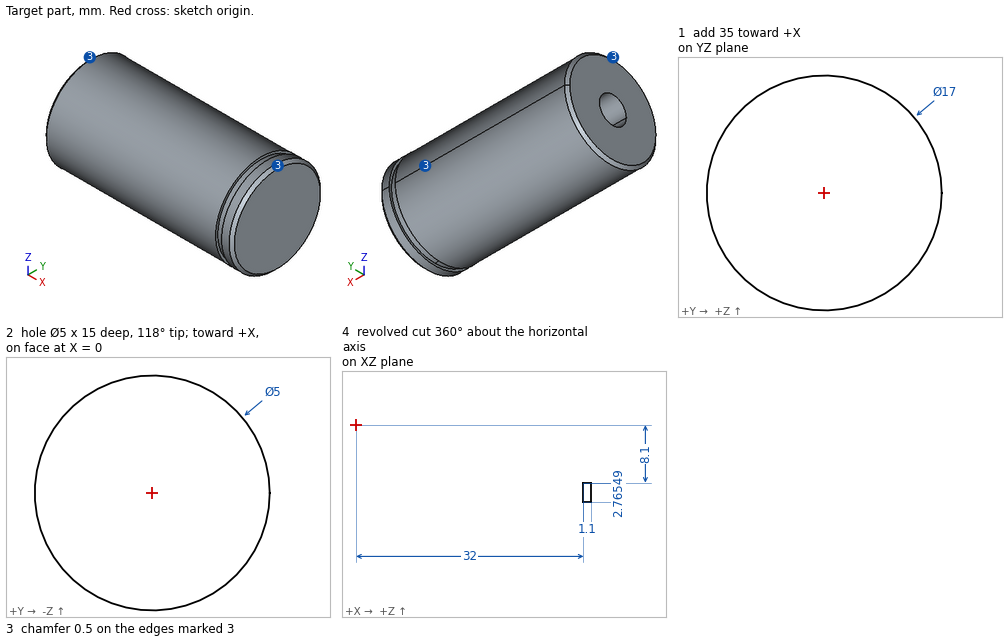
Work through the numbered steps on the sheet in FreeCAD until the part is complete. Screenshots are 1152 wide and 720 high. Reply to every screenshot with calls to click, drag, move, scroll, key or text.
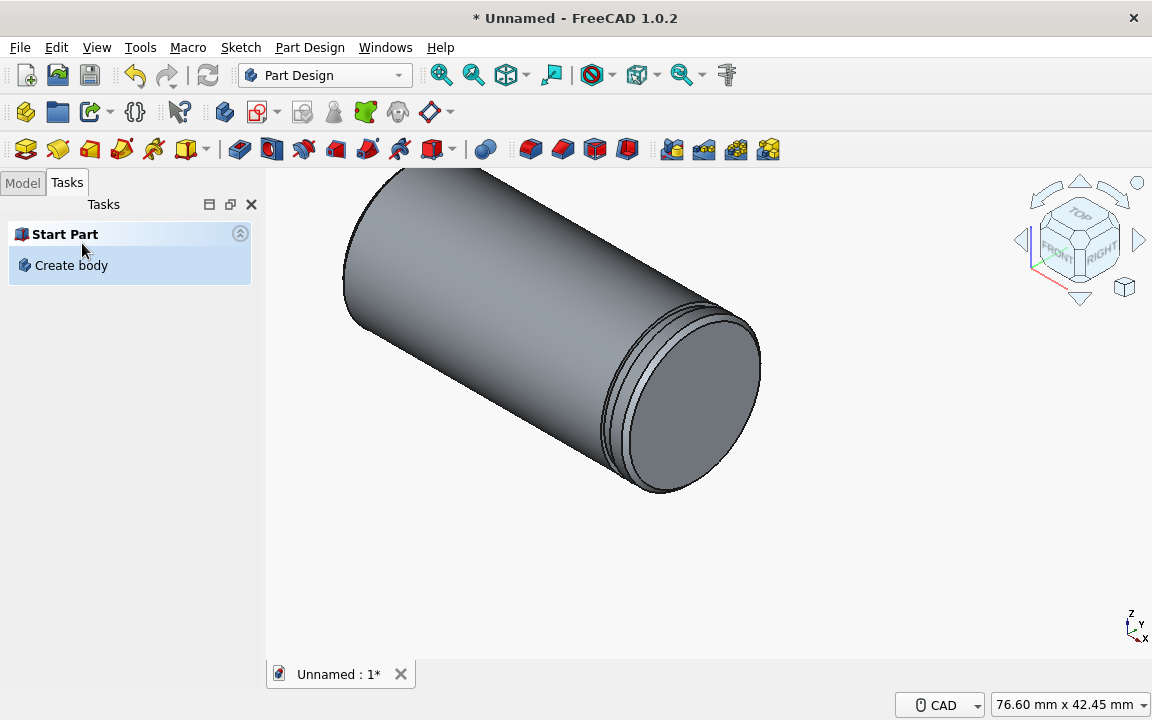
click(442, 76)